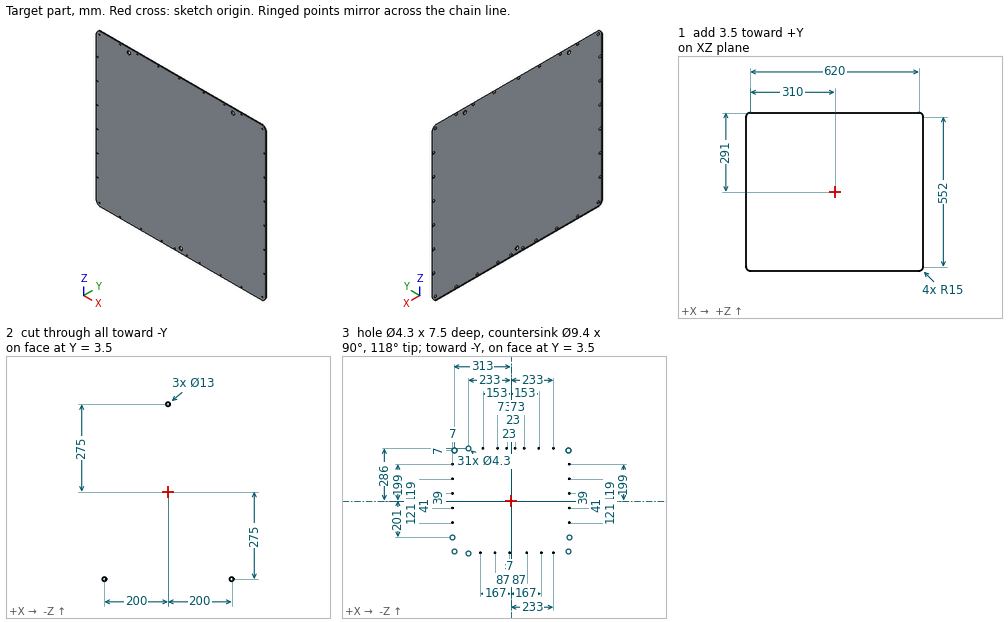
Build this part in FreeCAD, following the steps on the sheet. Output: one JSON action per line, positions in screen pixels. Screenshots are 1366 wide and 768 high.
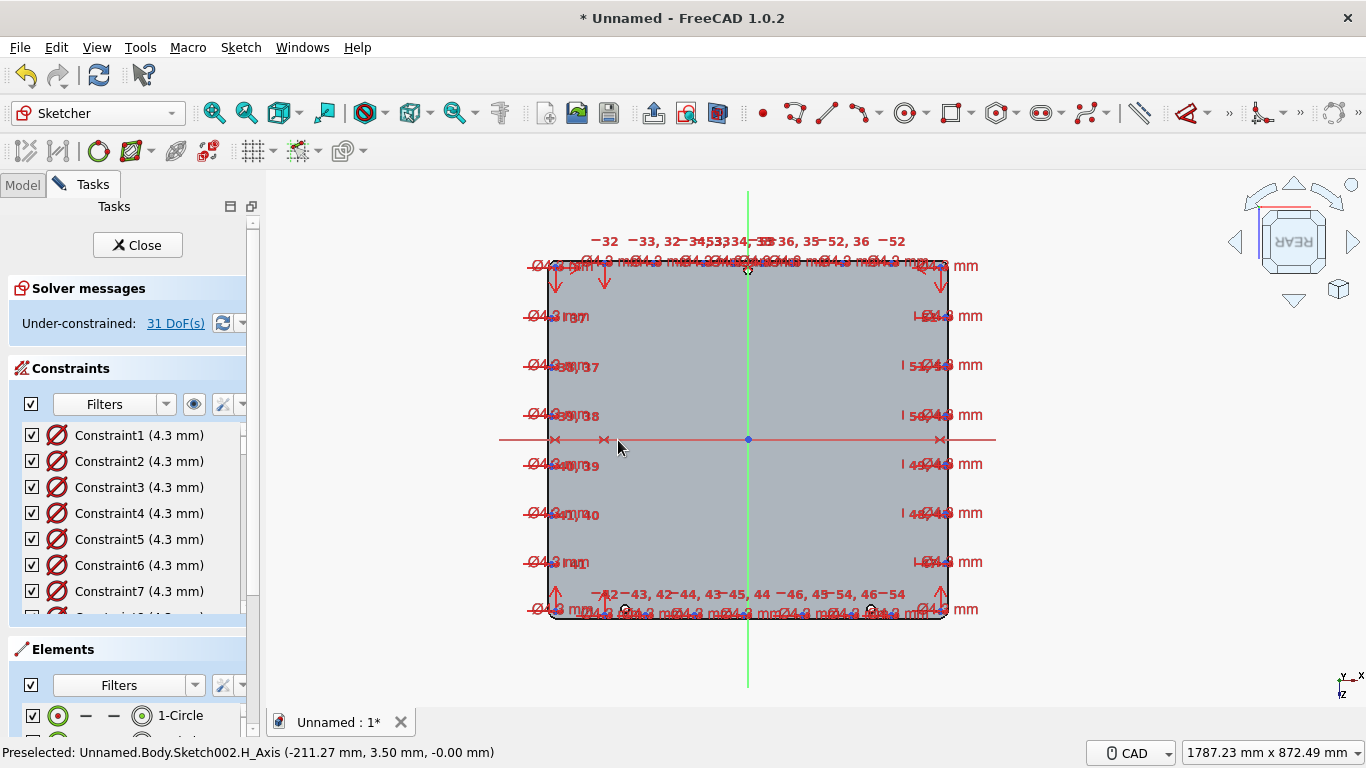
{"action": "left_click", "coordinate": [552, 564]}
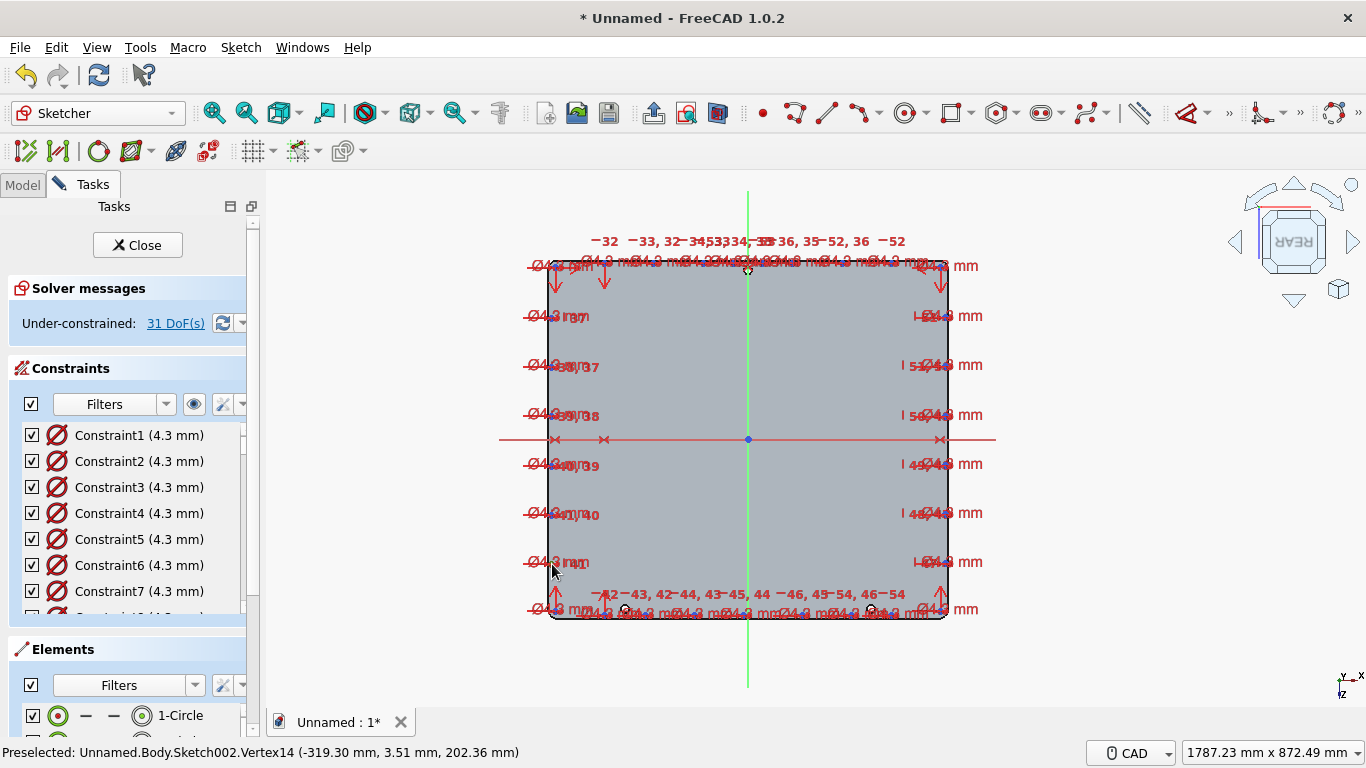
{"action": "left_click", "coordinate": [945, 564]}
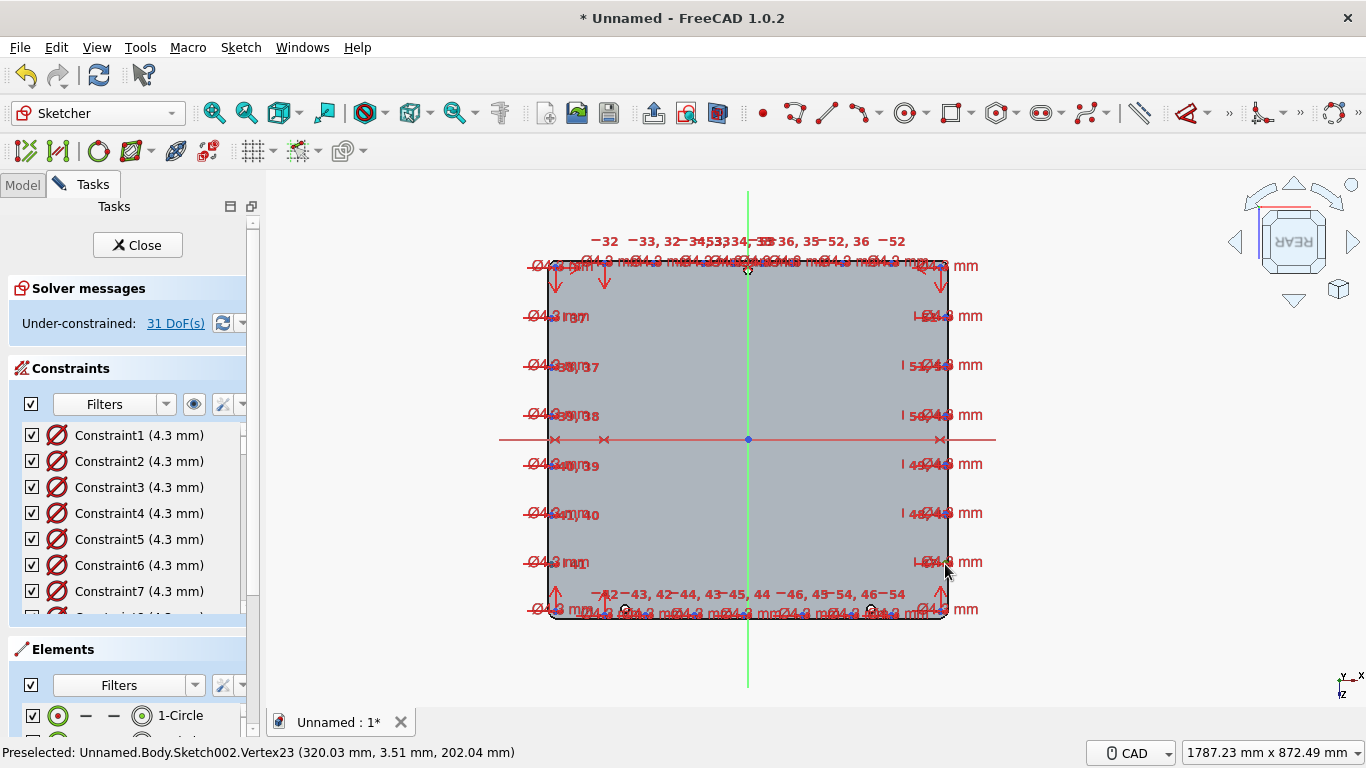
{"action": "left_click", "coordinate": [748, 576]}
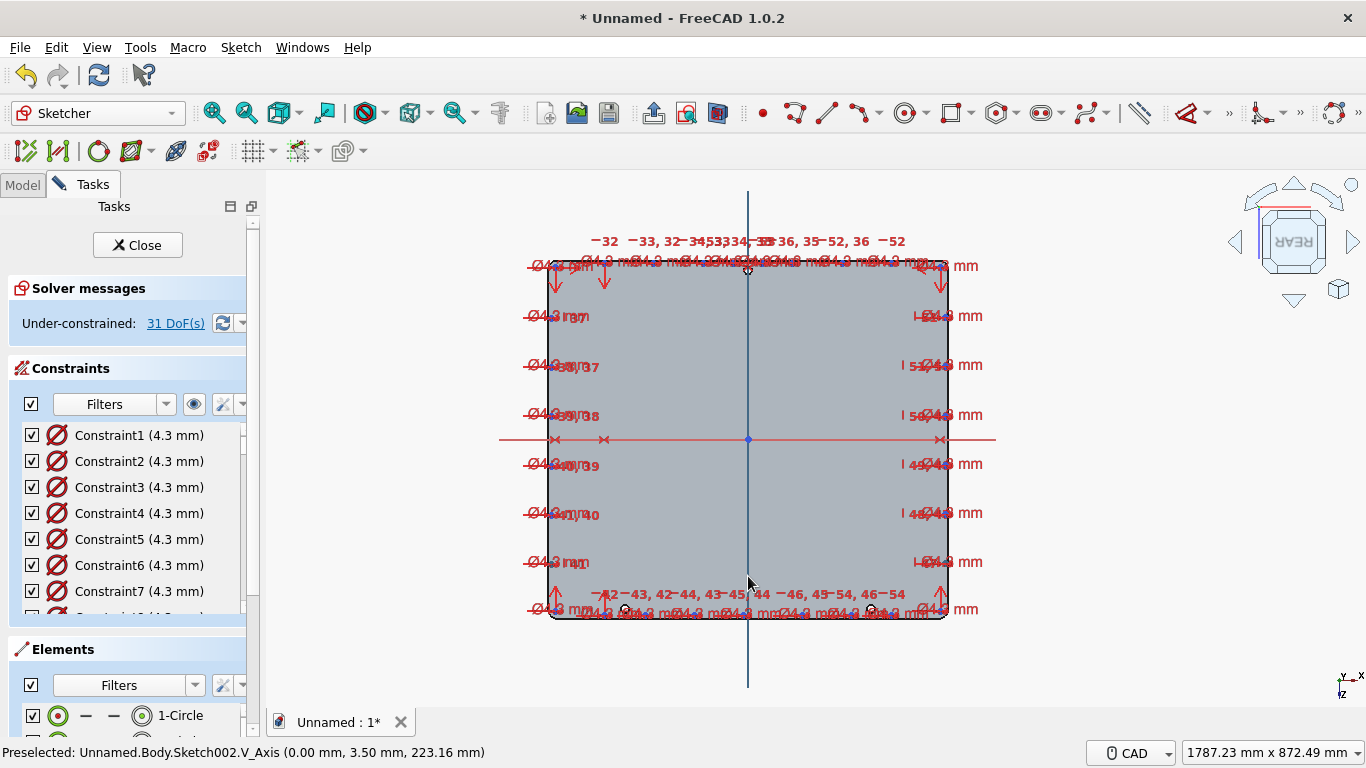
{"action": "key", "text": "s"}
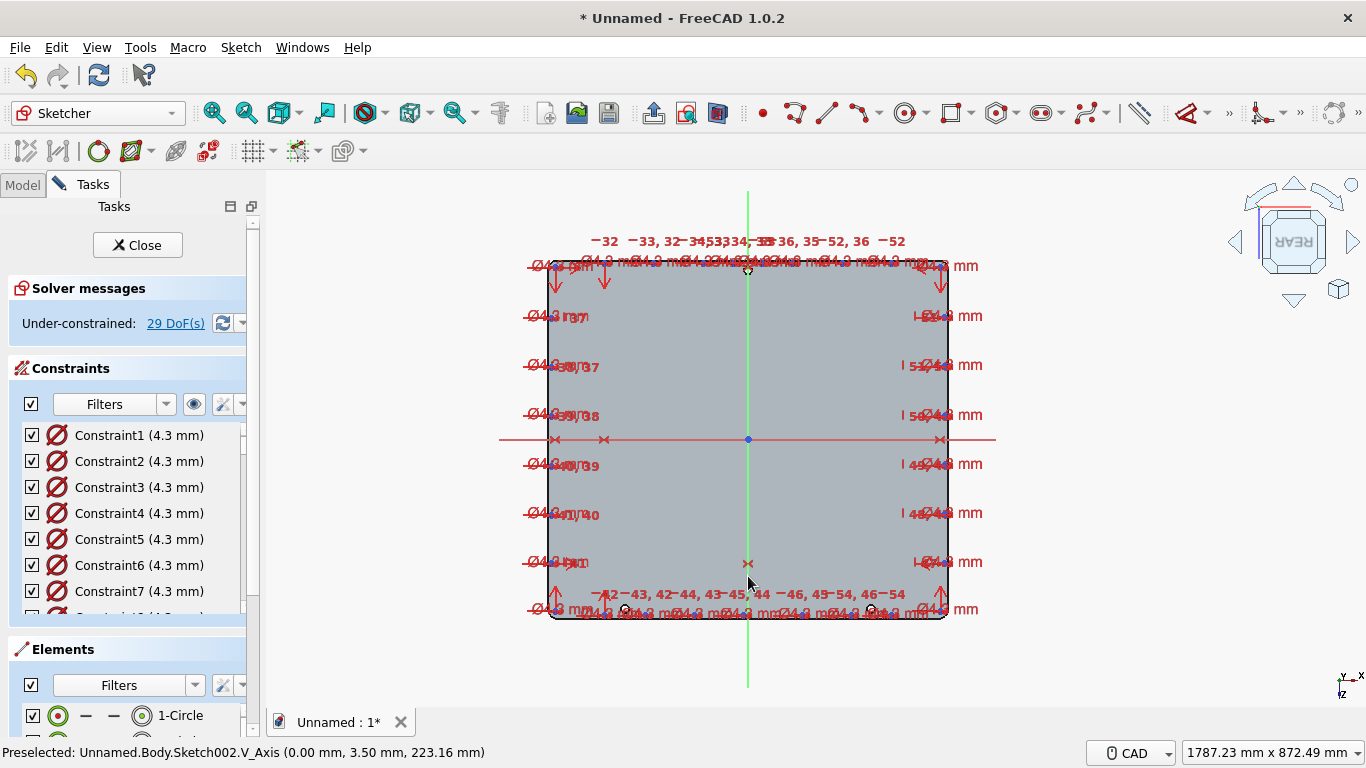
{"action": "left_click", "coordinate": [1186, 114]}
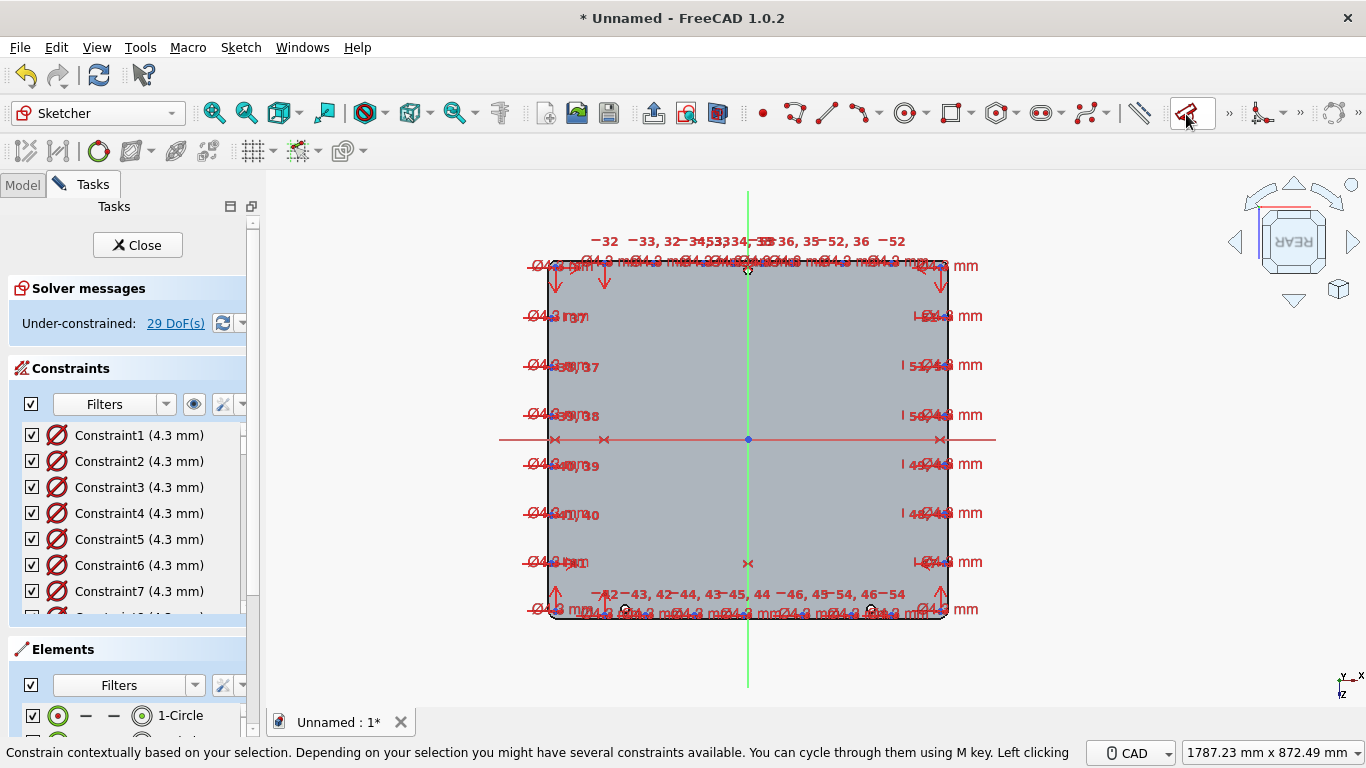
{"action": "scroll", "coordinate": [744, 616], "scroll_direction": "up", "scroll_amount": 12}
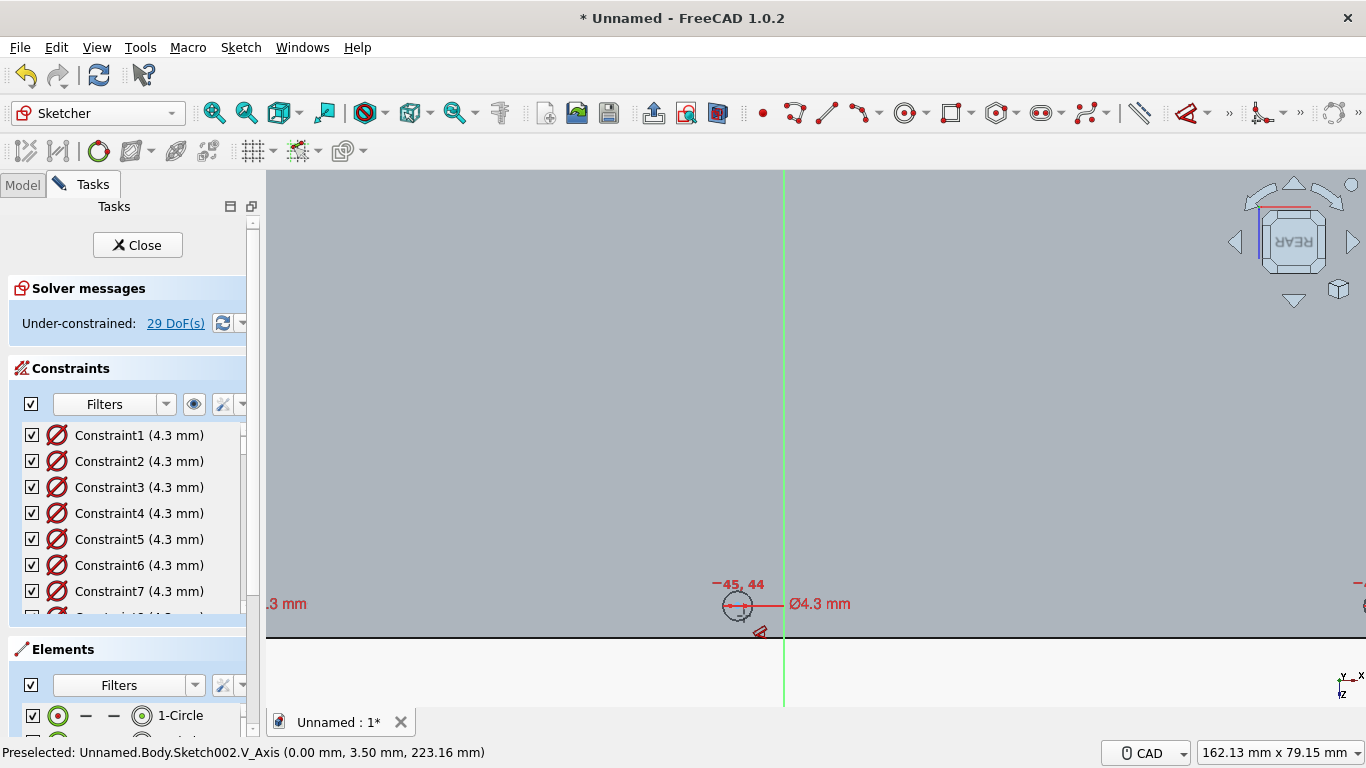
{"action": "left_click", "coordinate": [738, 606]}
{"action": "left_click", "coordinate": [761, 640]}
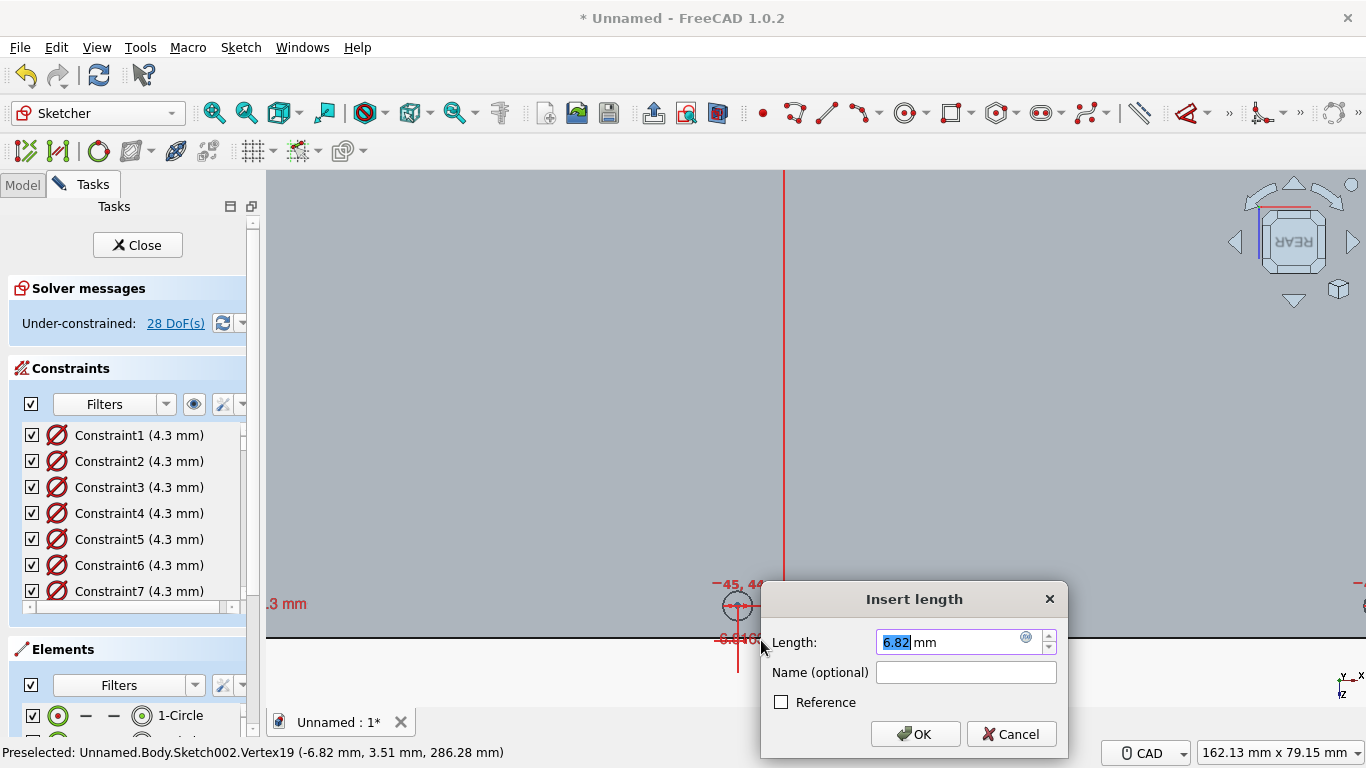
{"action": "type", "text": "7"}
{"action": "key", "text": "Return"}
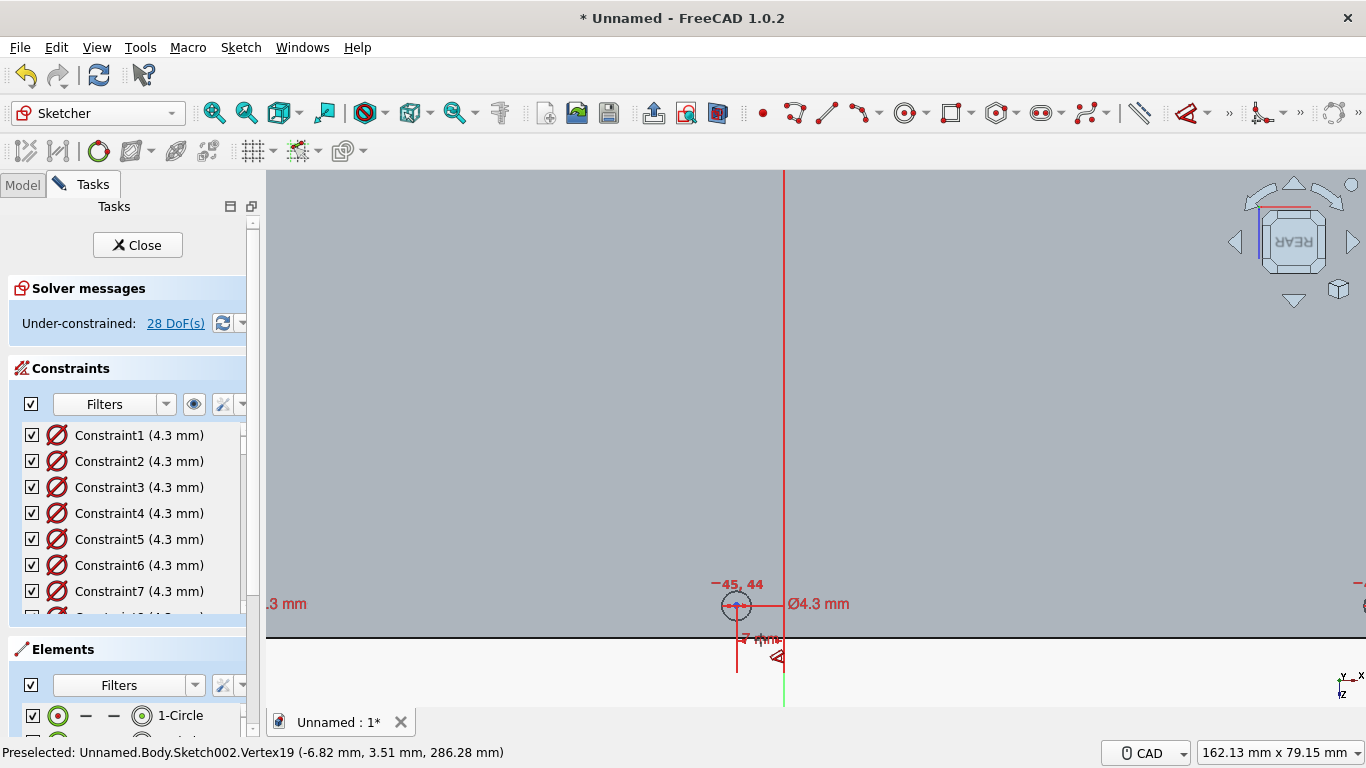
{"action": "scroll", "coordinate": [744, 616], "scroll_direction": "down", "scroll_amount": 12}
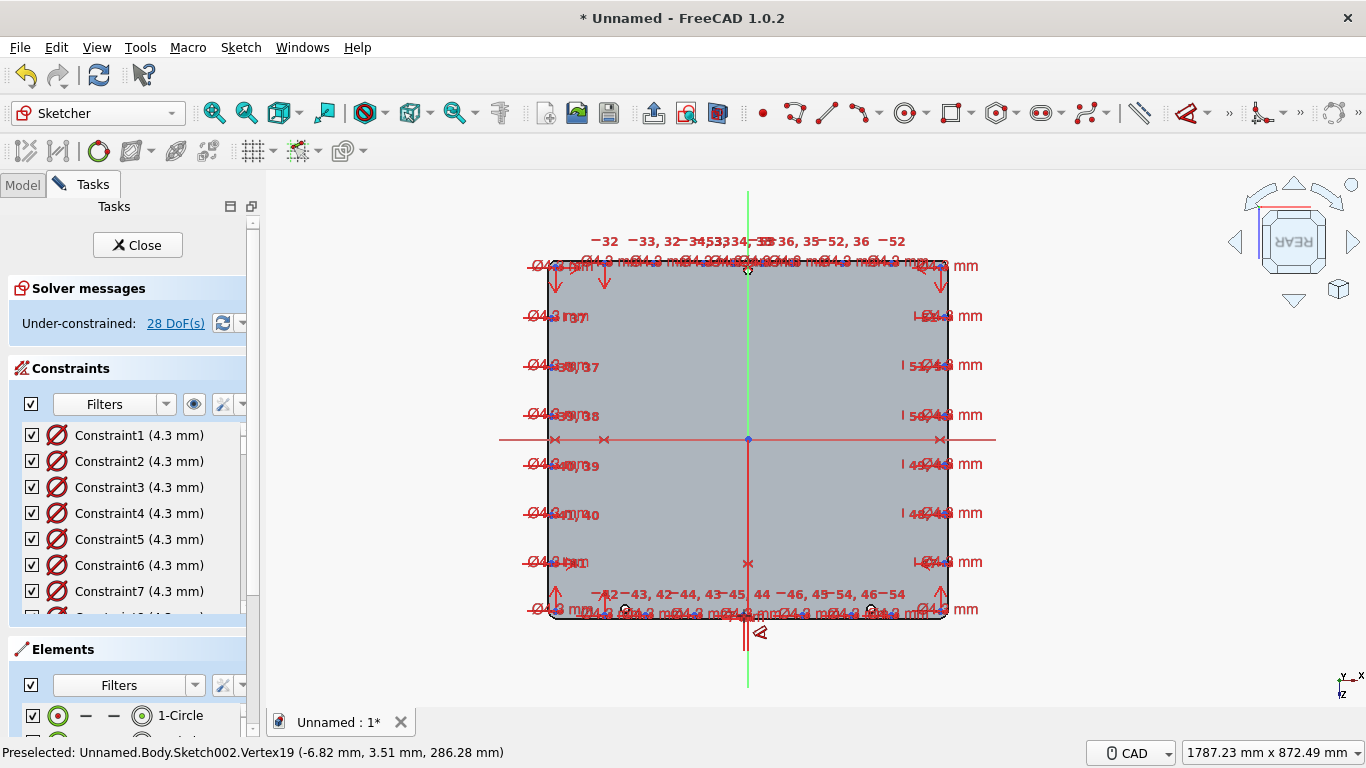
{"action": "left_click", "coordinate": [704, 263]}
{"action": "left_click", "coordinate": [726, 229]}